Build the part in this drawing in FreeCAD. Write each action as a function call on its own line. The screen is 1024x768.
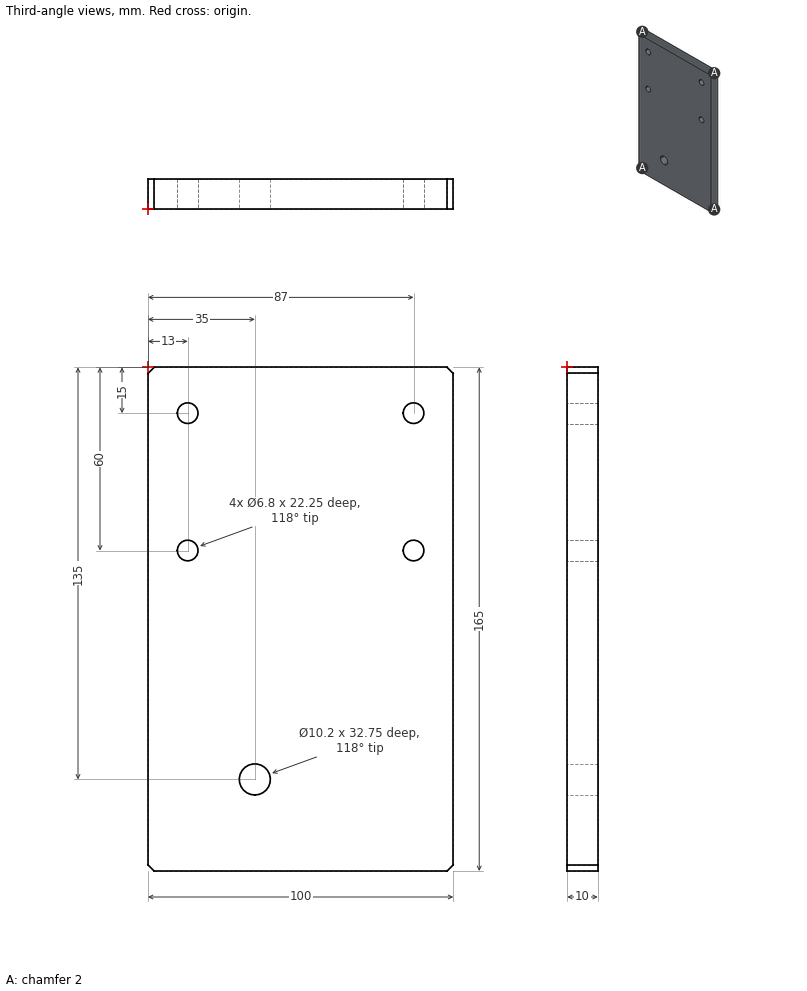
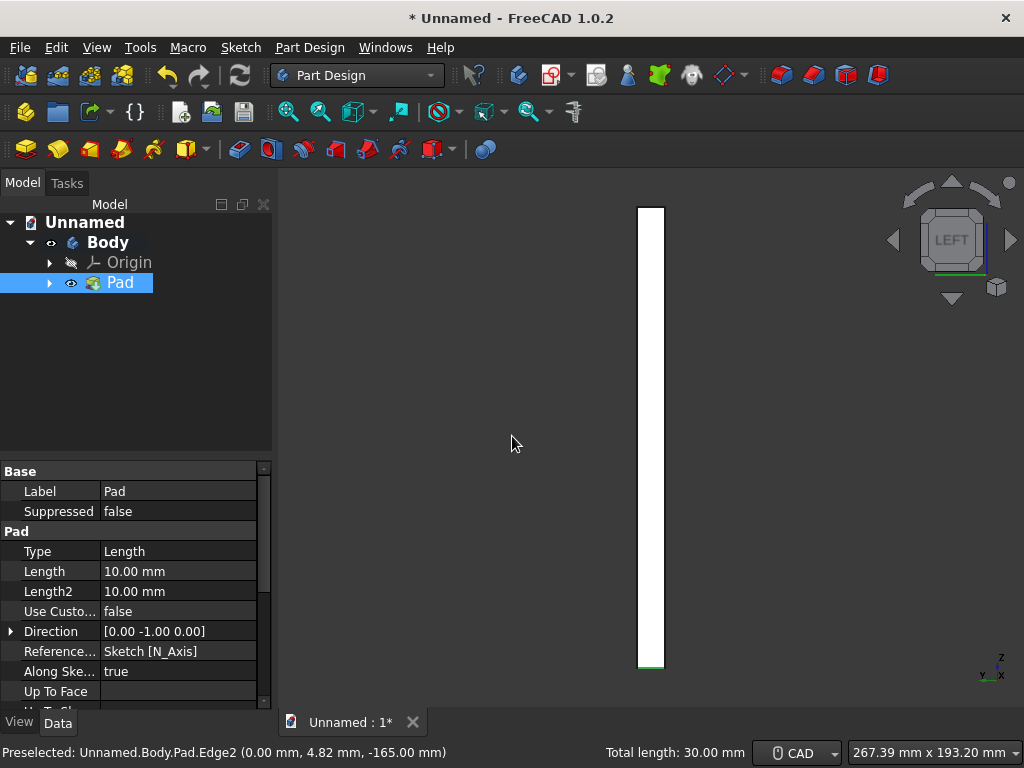
key(v)
key(3)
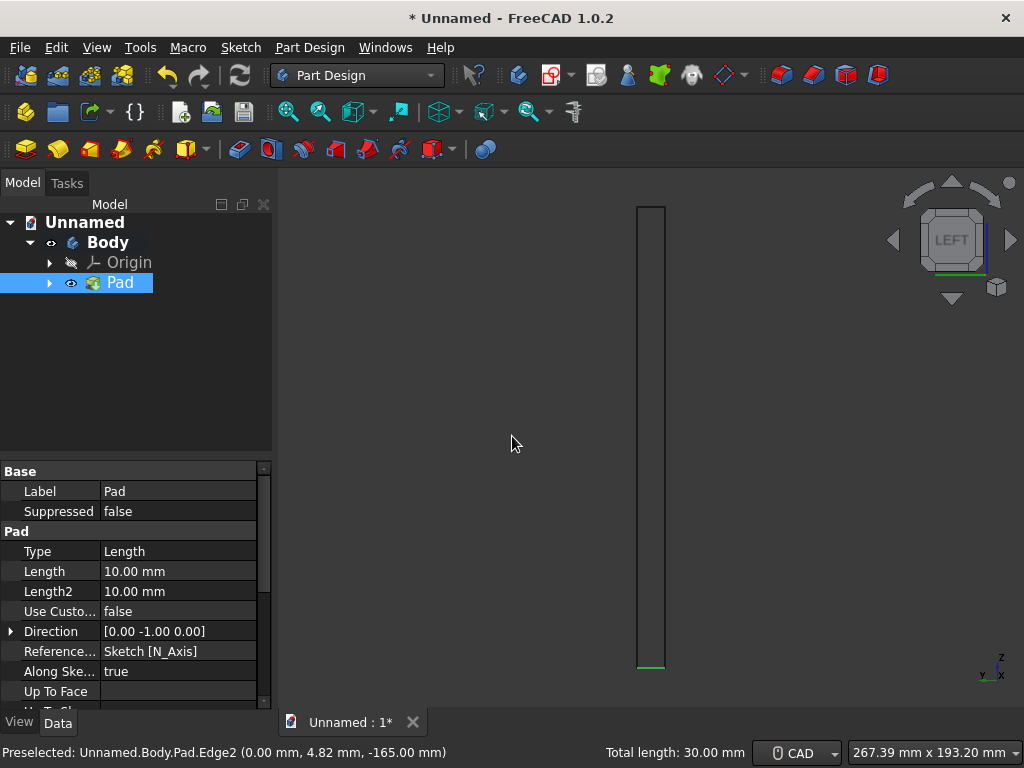
key(0)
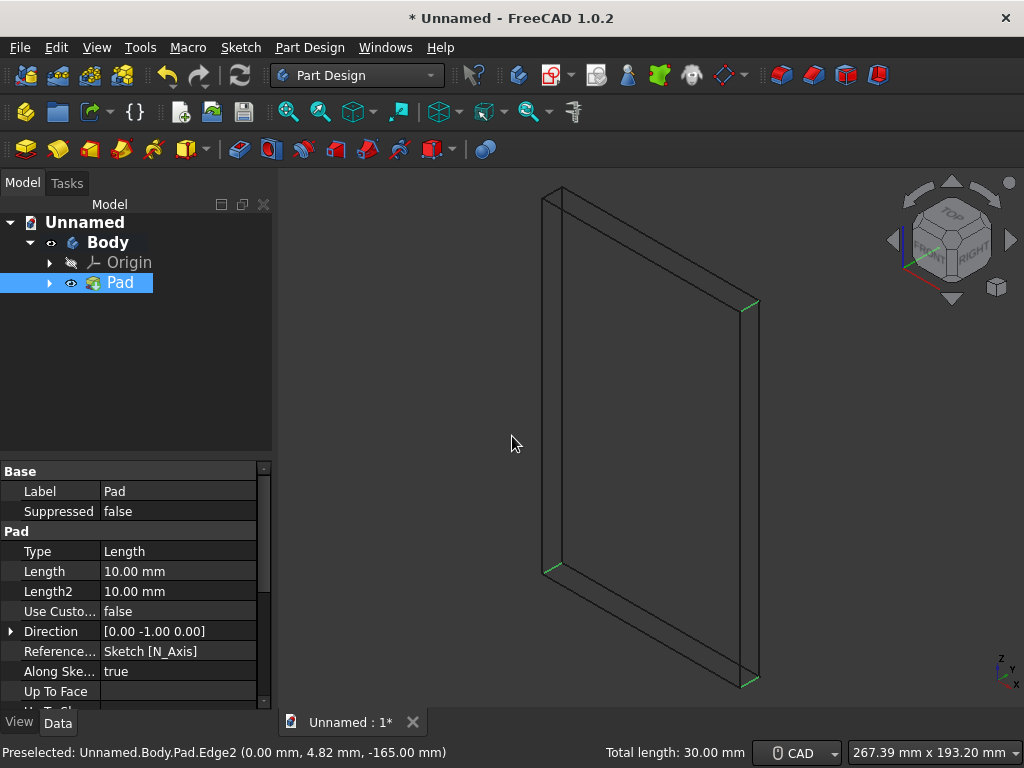
key(2)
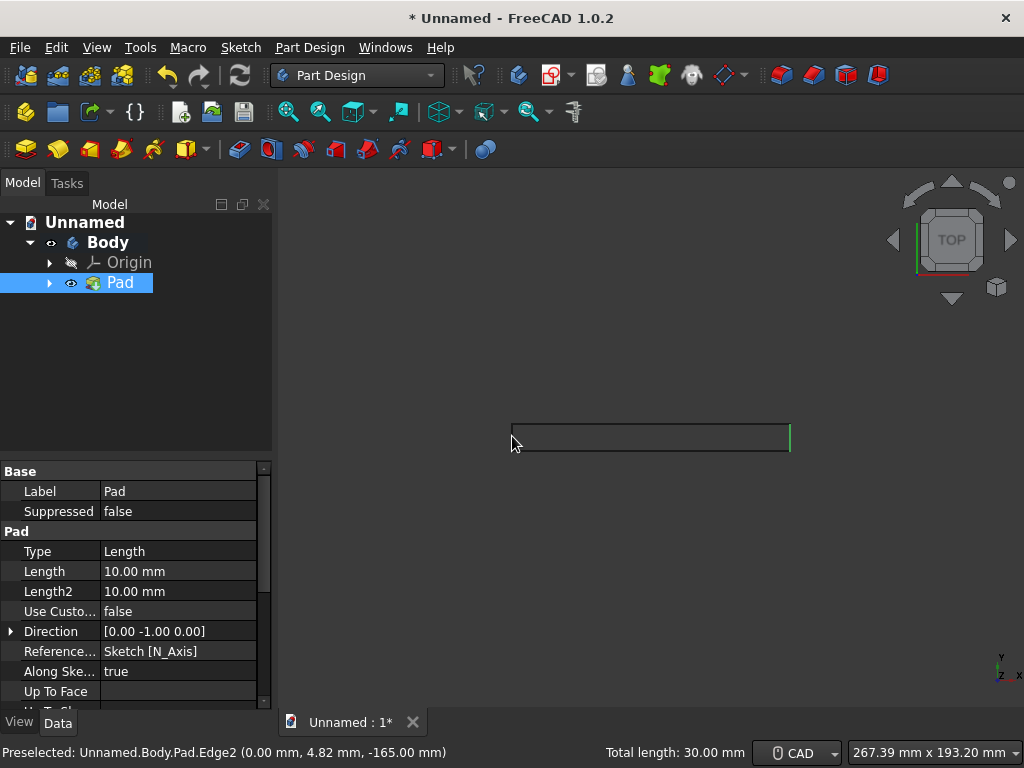
click(290, 112)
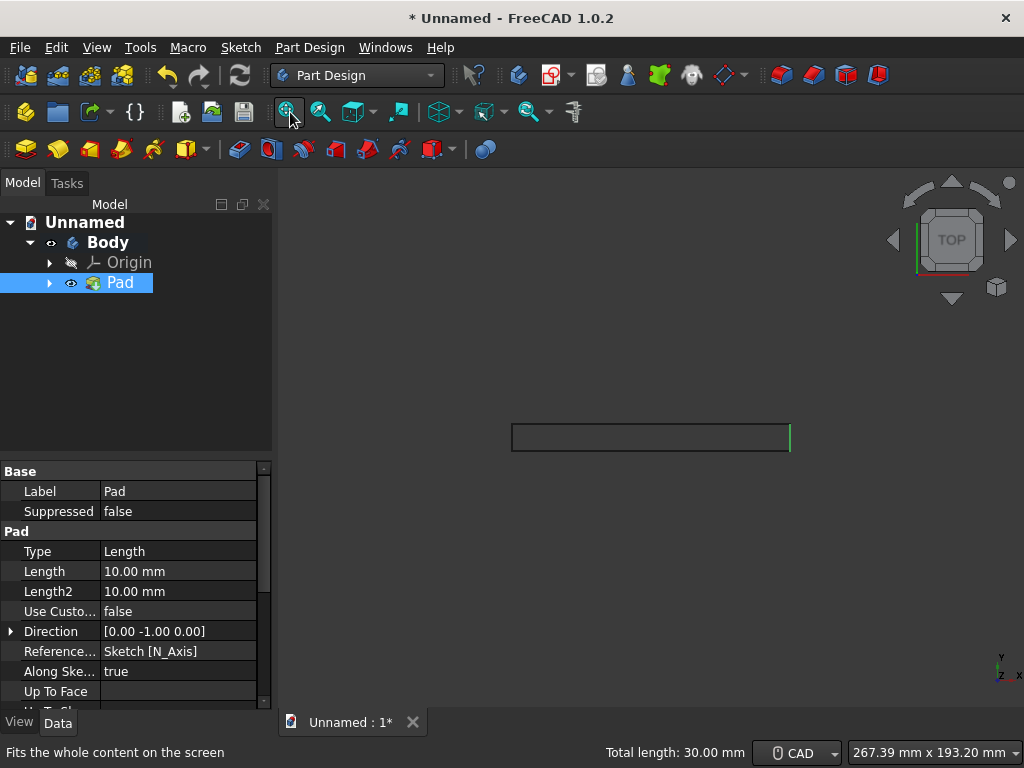
click(512, 437, ctrl)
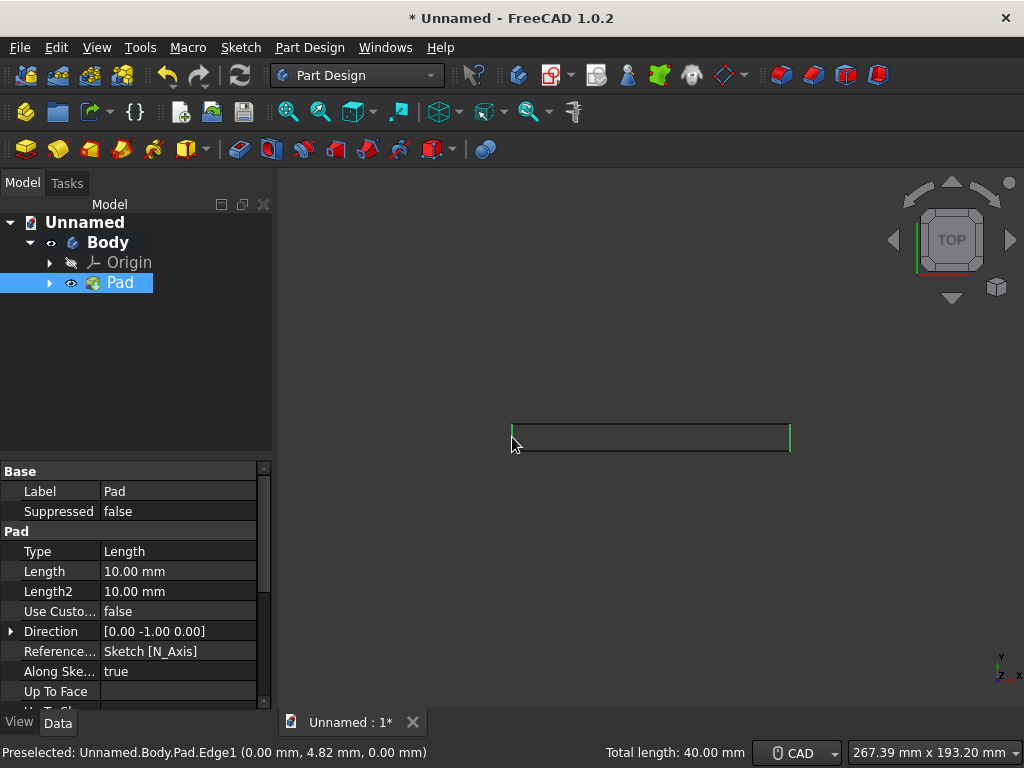
key(v)
key(1)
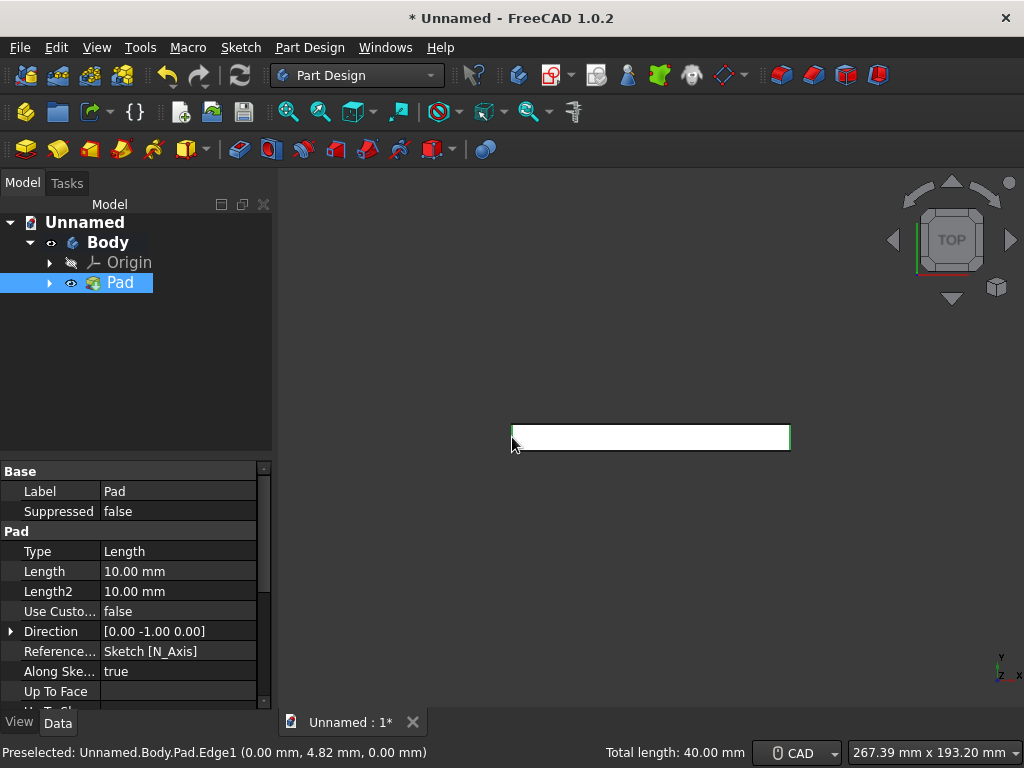
click(814, 76)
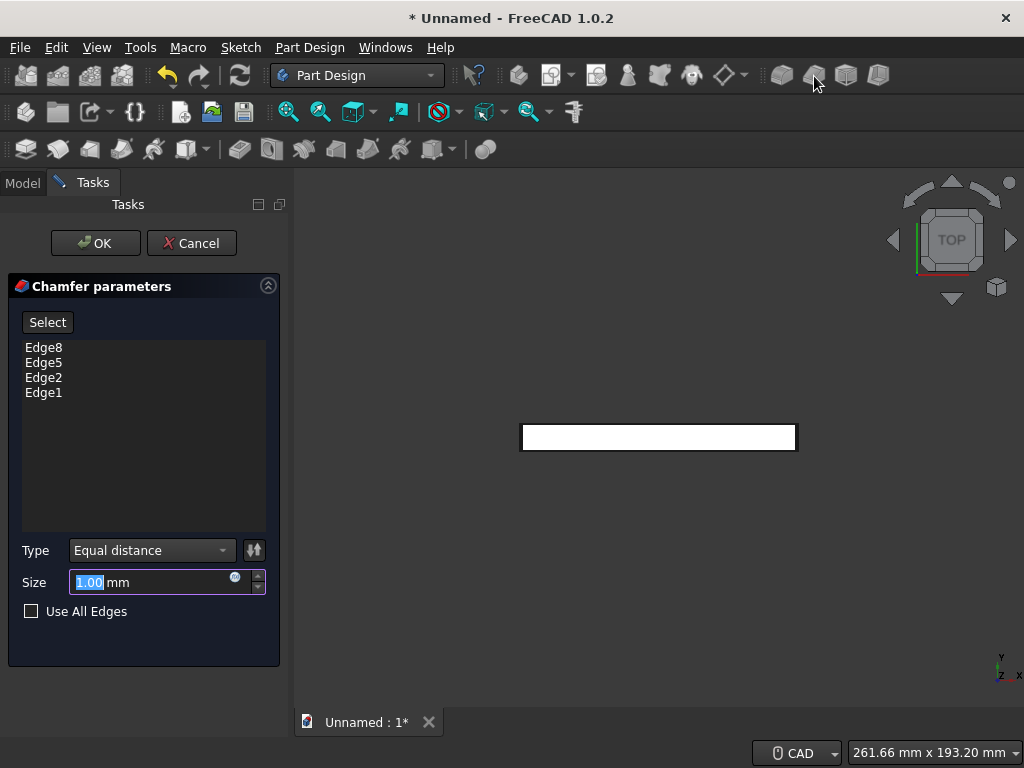
text(2)
key(Tab)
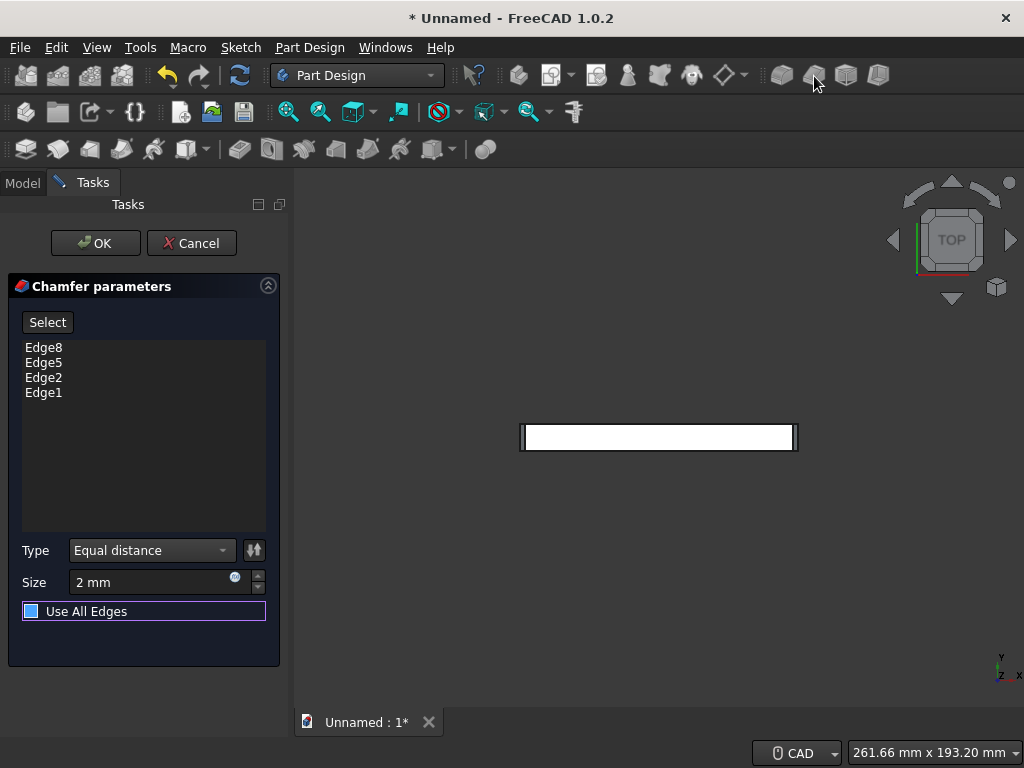
click(96, 243)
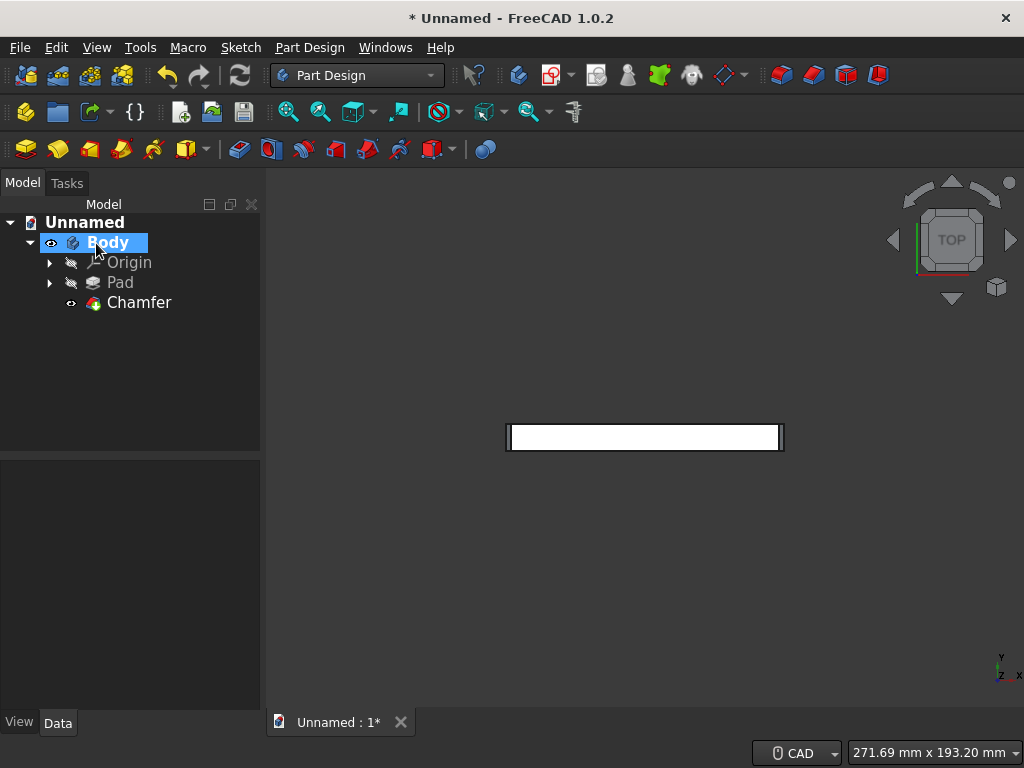
click(290, 112)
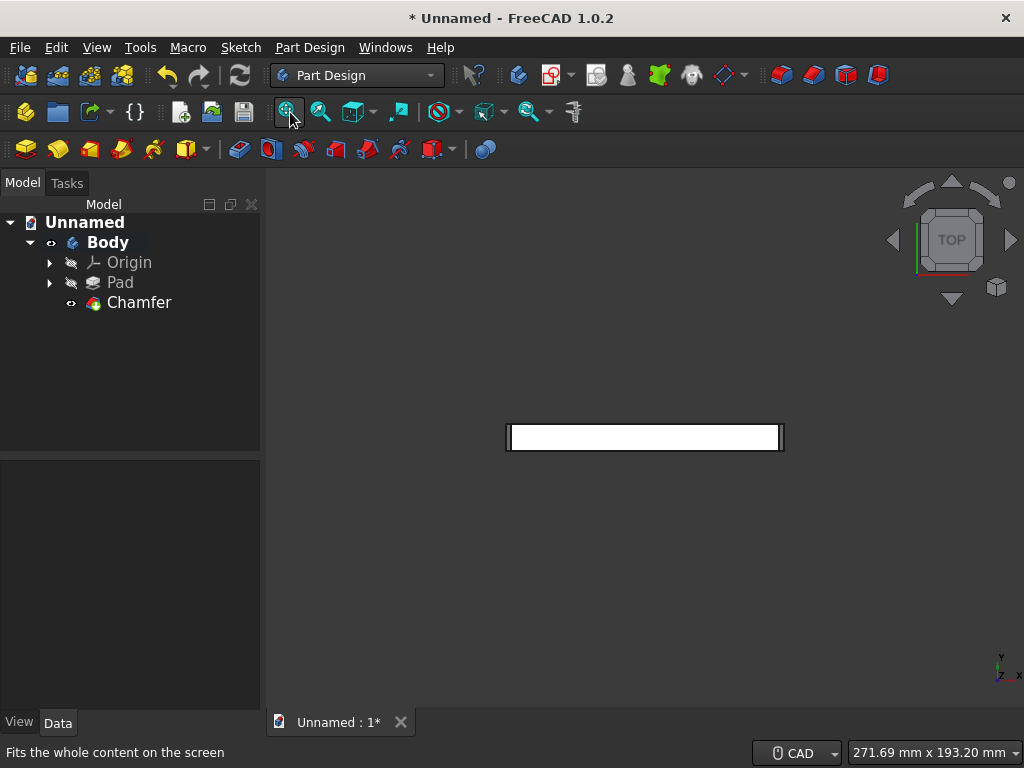
key(4)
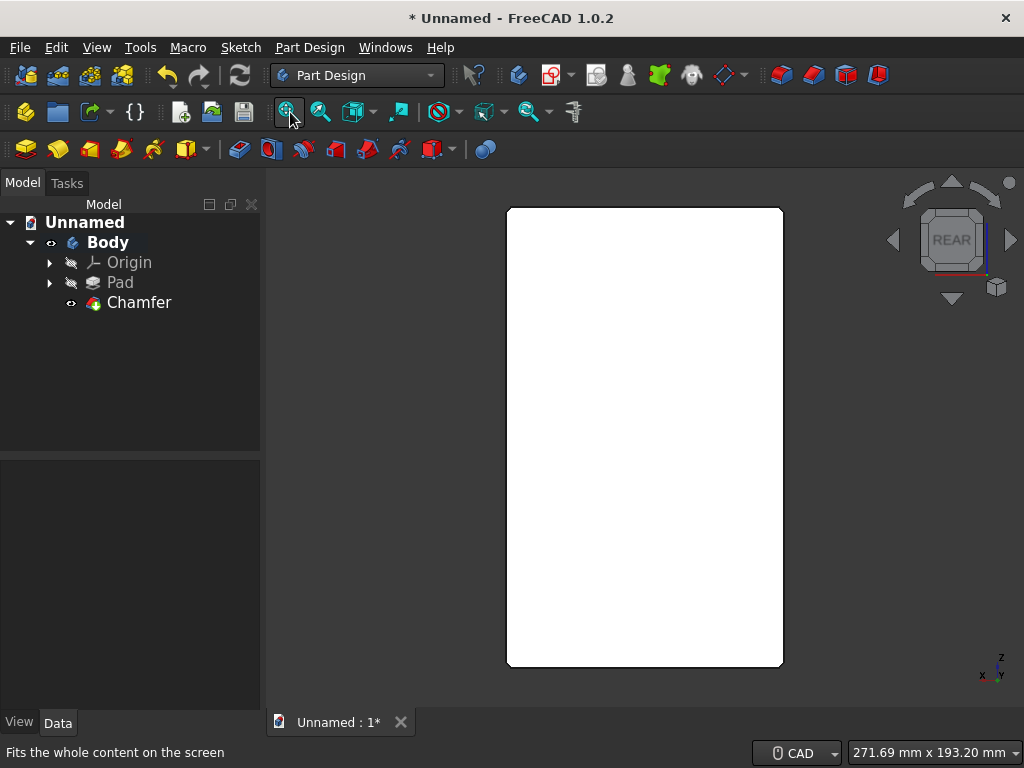
click(645, 371)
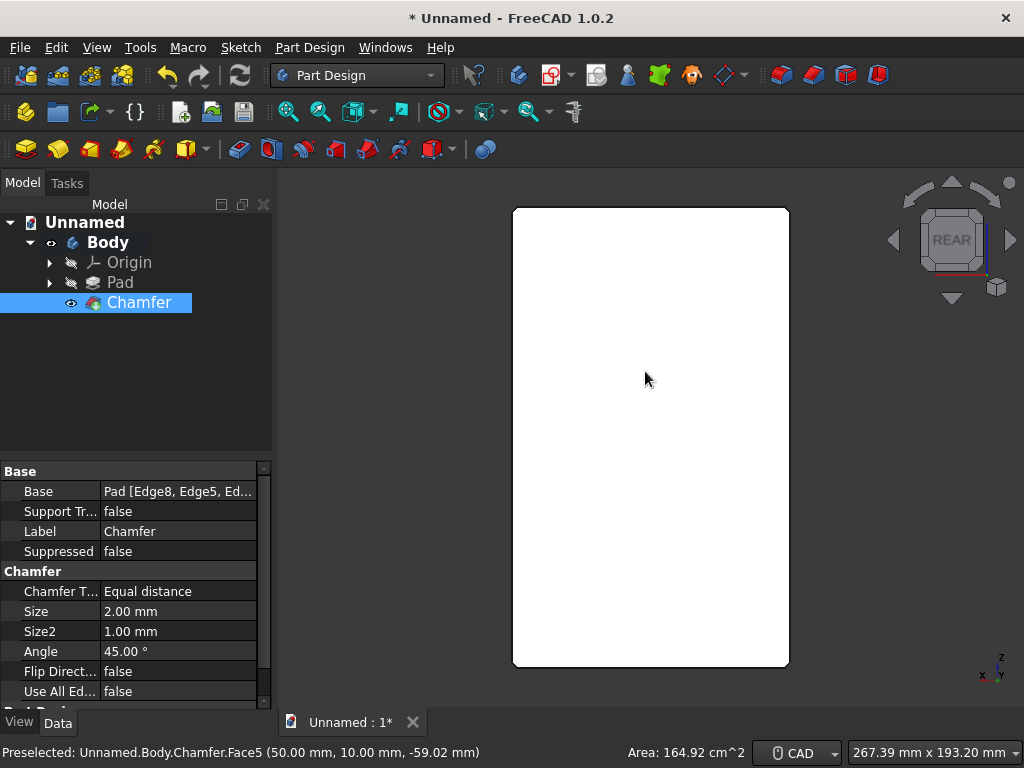
click(552, 76)